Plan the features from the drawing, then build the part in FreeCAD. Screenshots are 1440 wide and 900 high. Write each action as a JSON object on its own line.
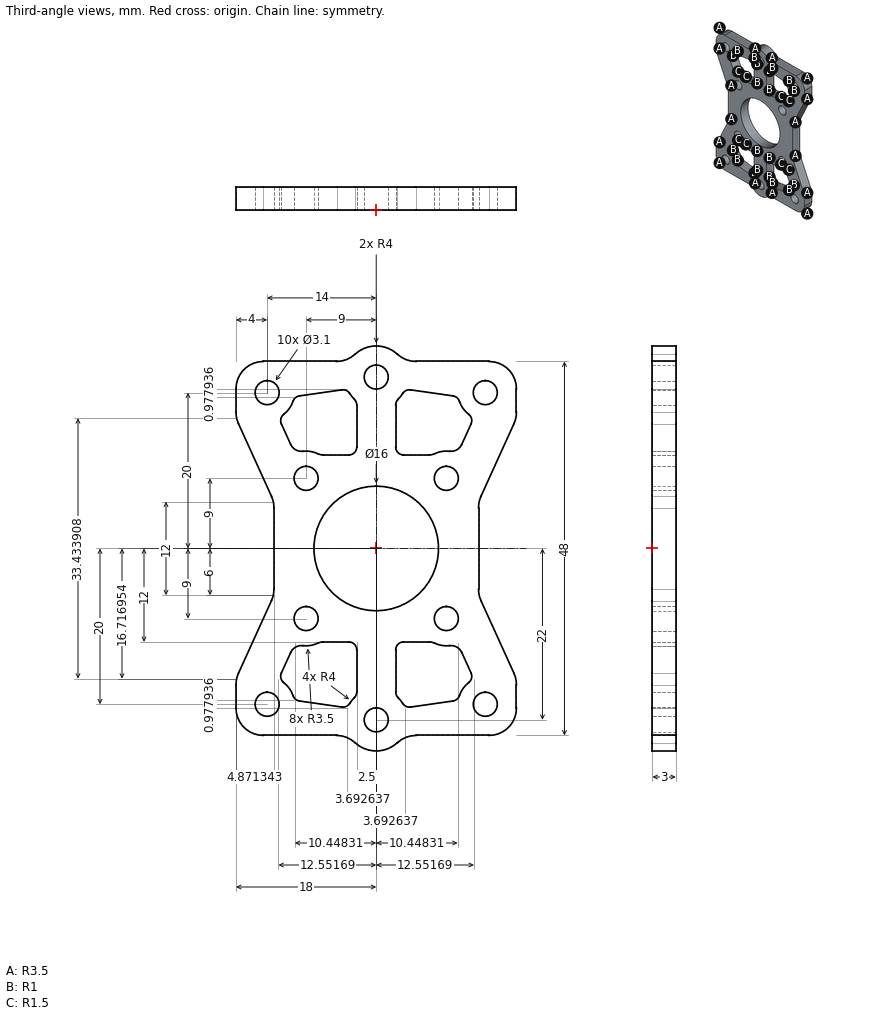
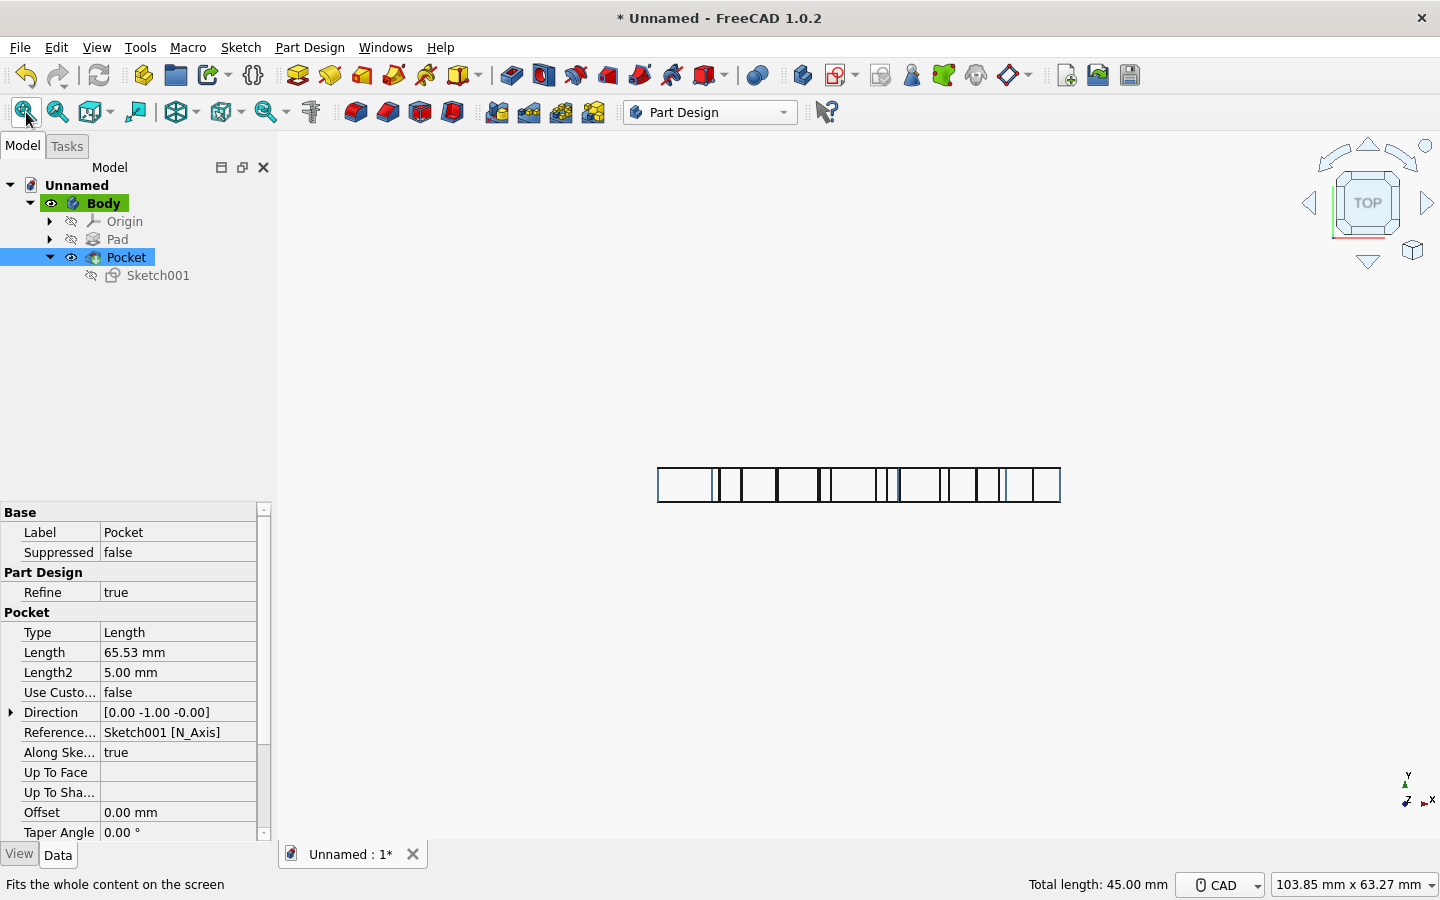
{"action": "left_click", "coordinate": [820, 484], "text": "ctrl"}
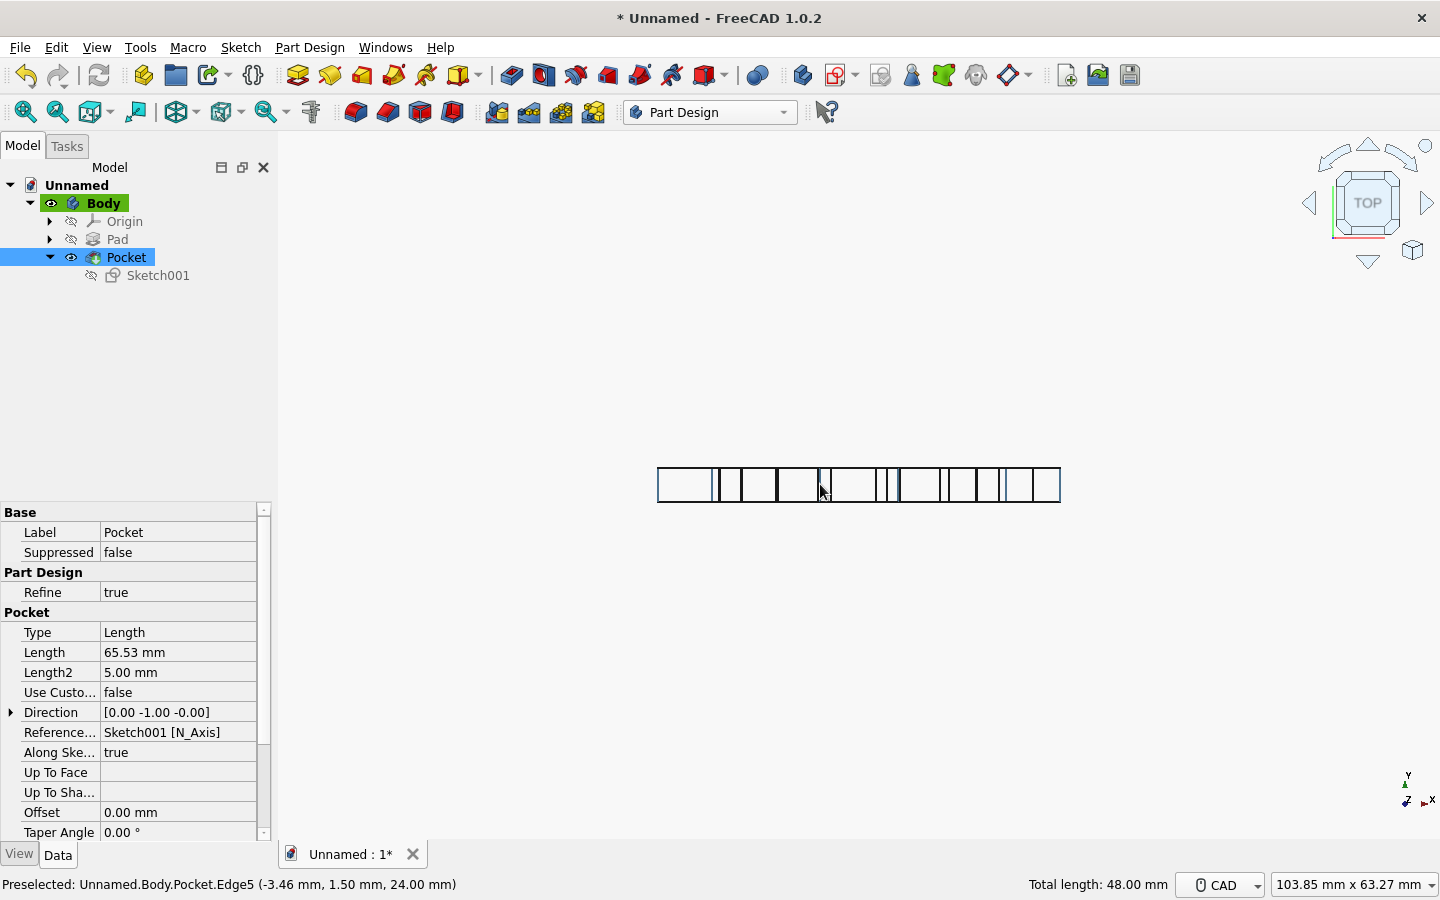
{"action": "key", "text": "v 1"}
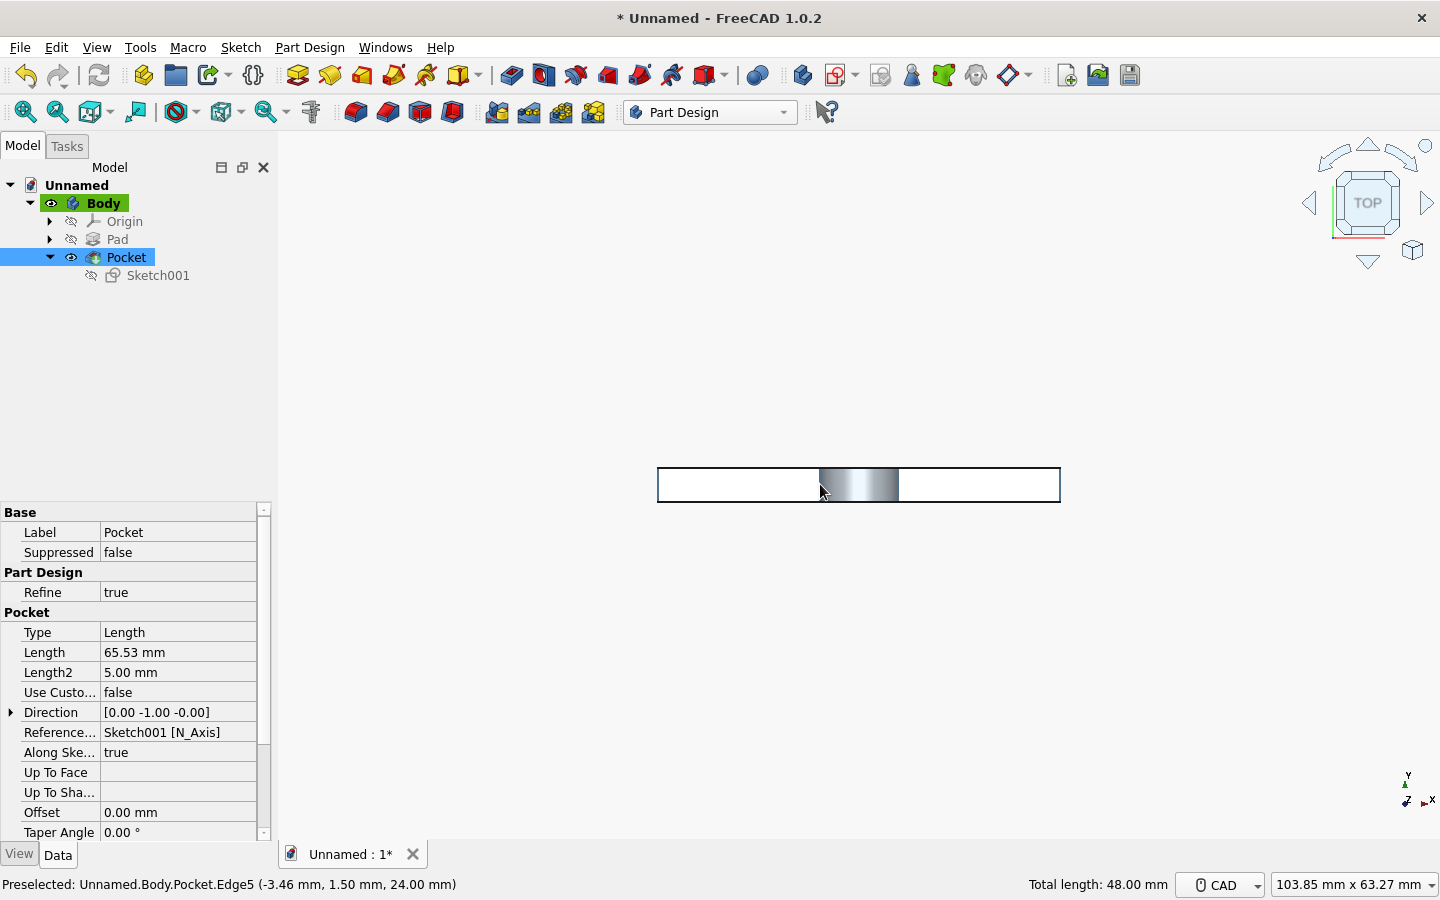
{"action": "left_click", "coordinate": [356, 112]}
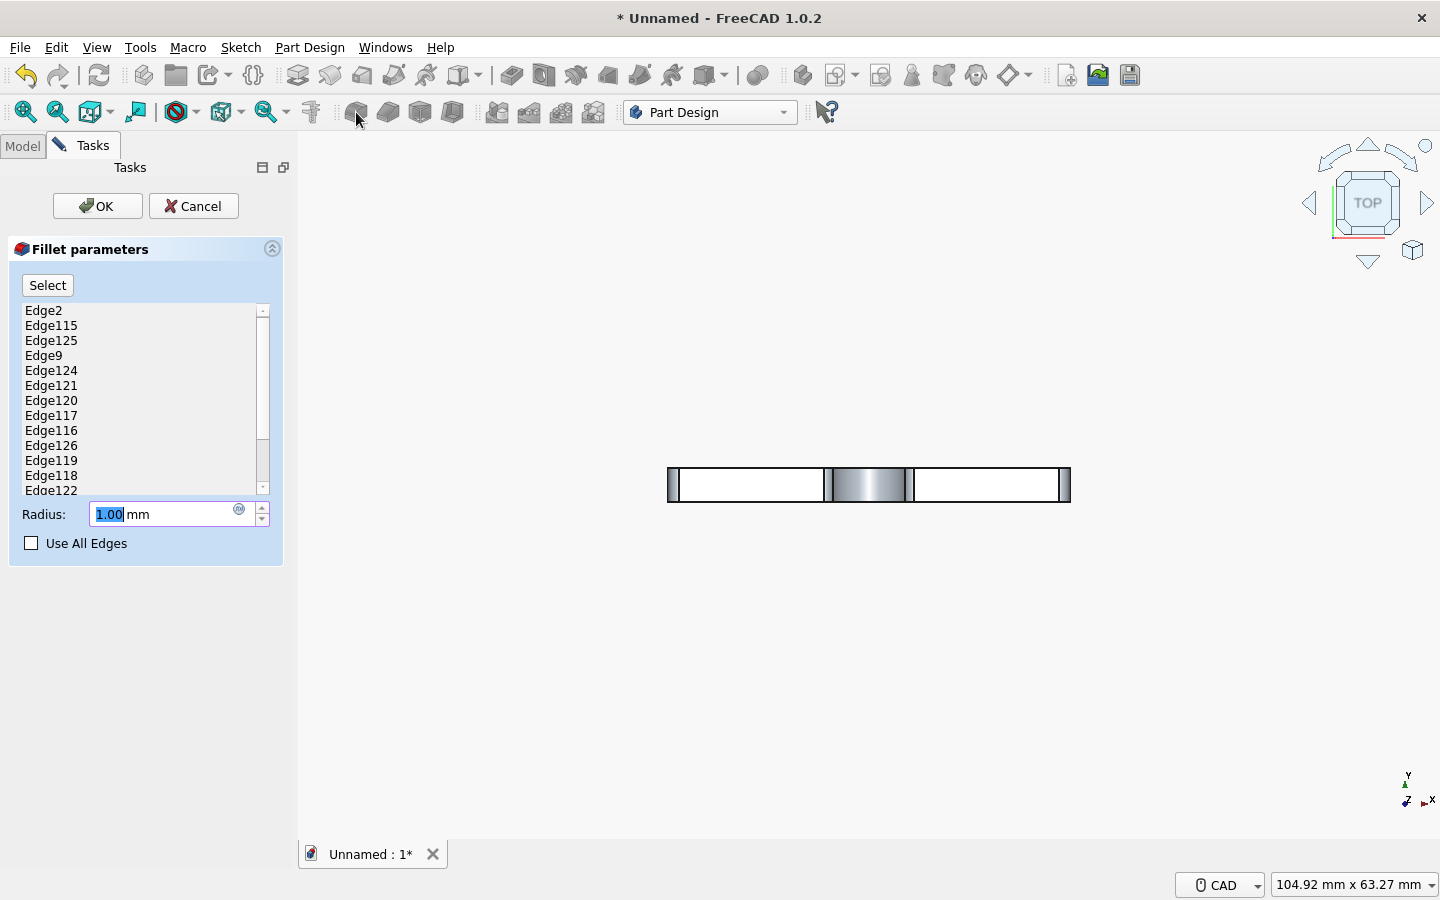
{"action": "type", "text": "3.5"}
{"action": "key", "text": "Tab"}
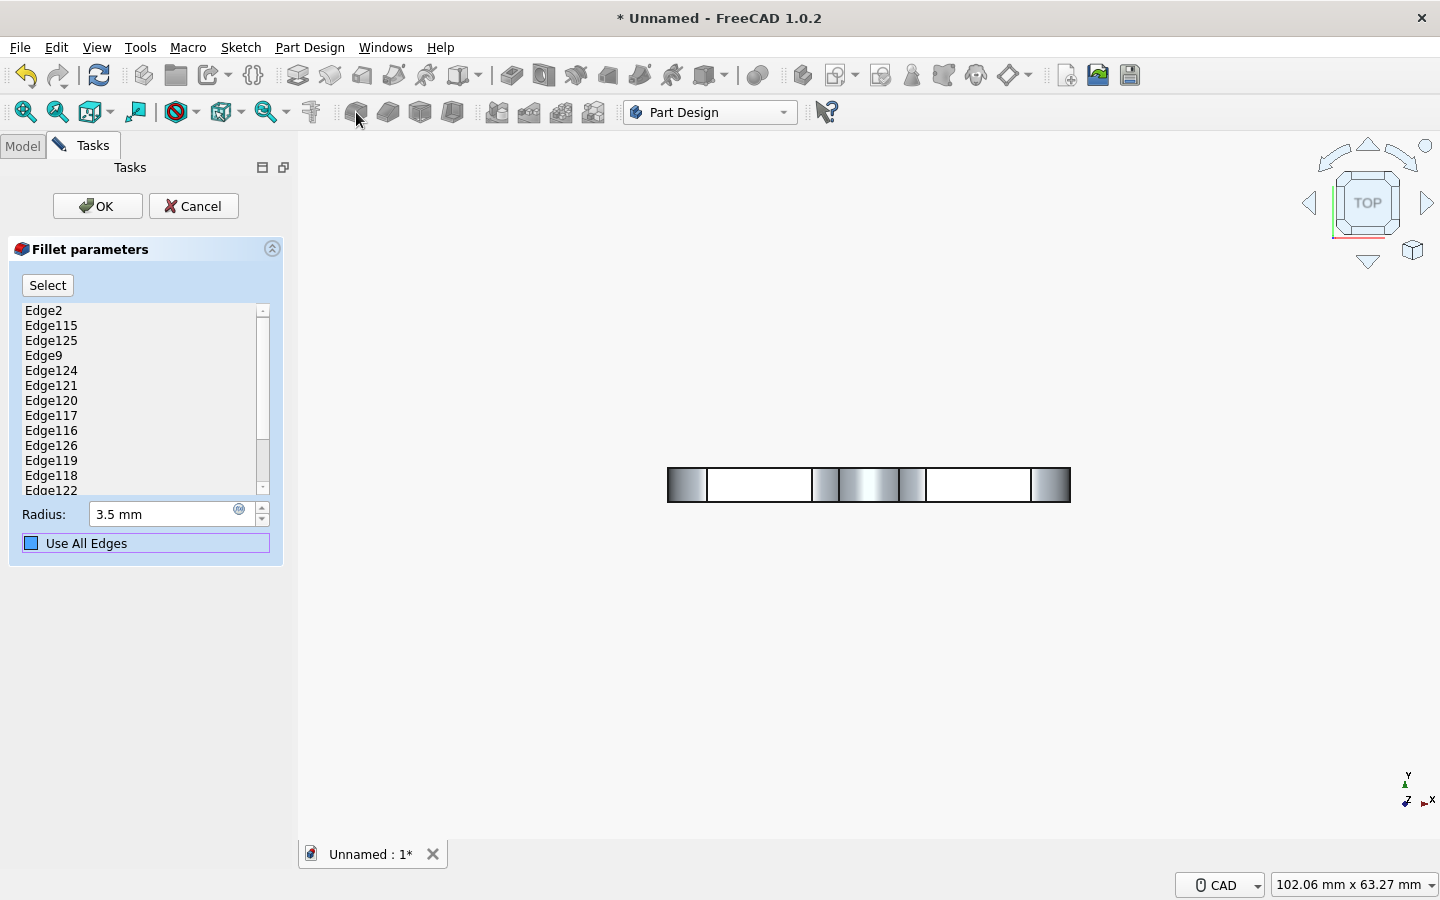
{"action": "left_click", "coordinate": [98, 206]}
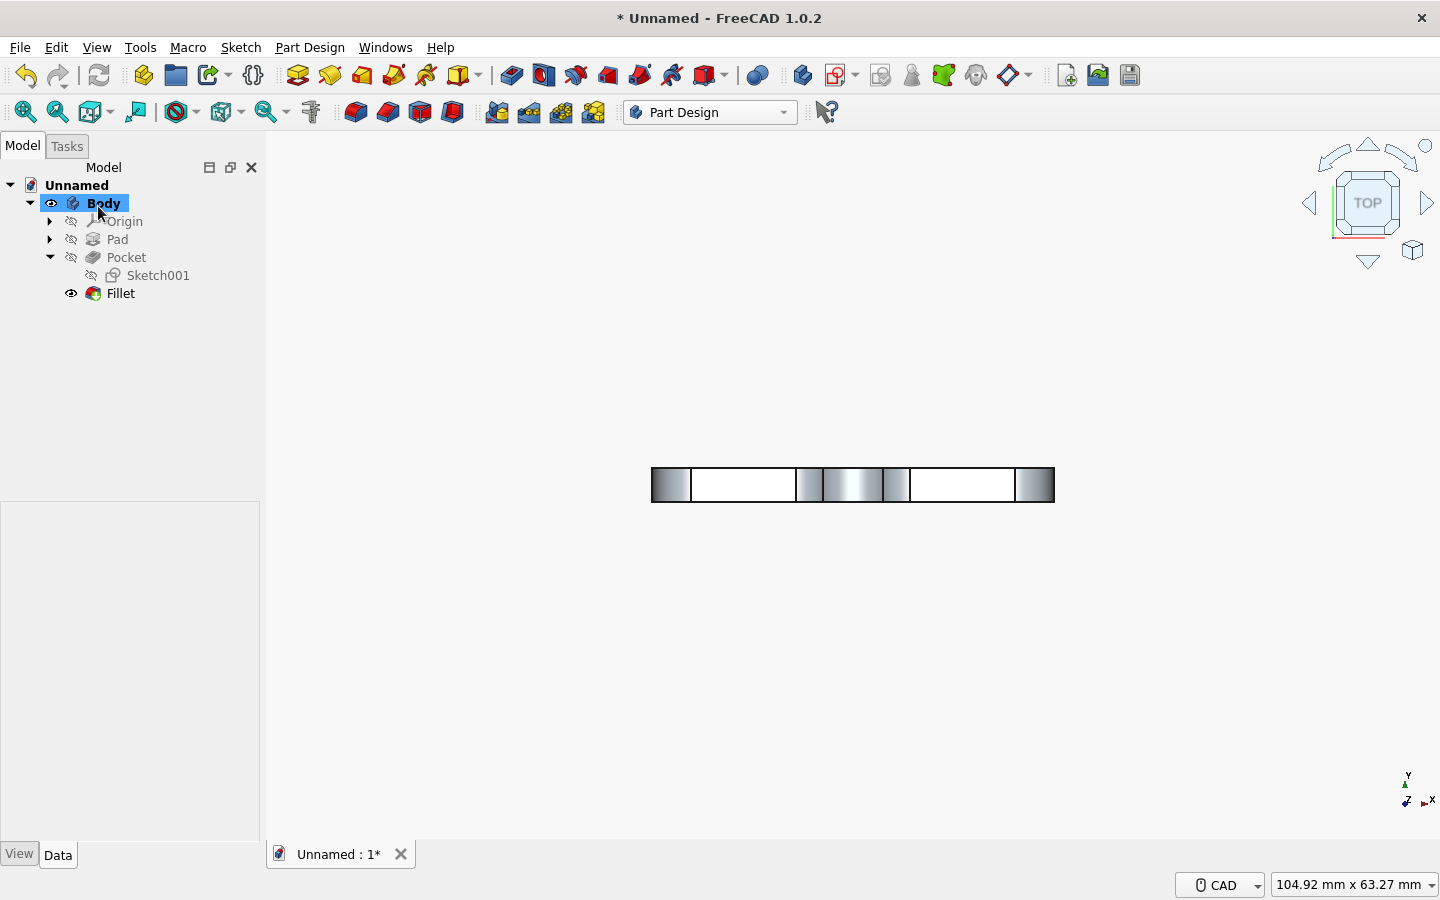
{"action": "left_click", "coordinate": [26, 112]}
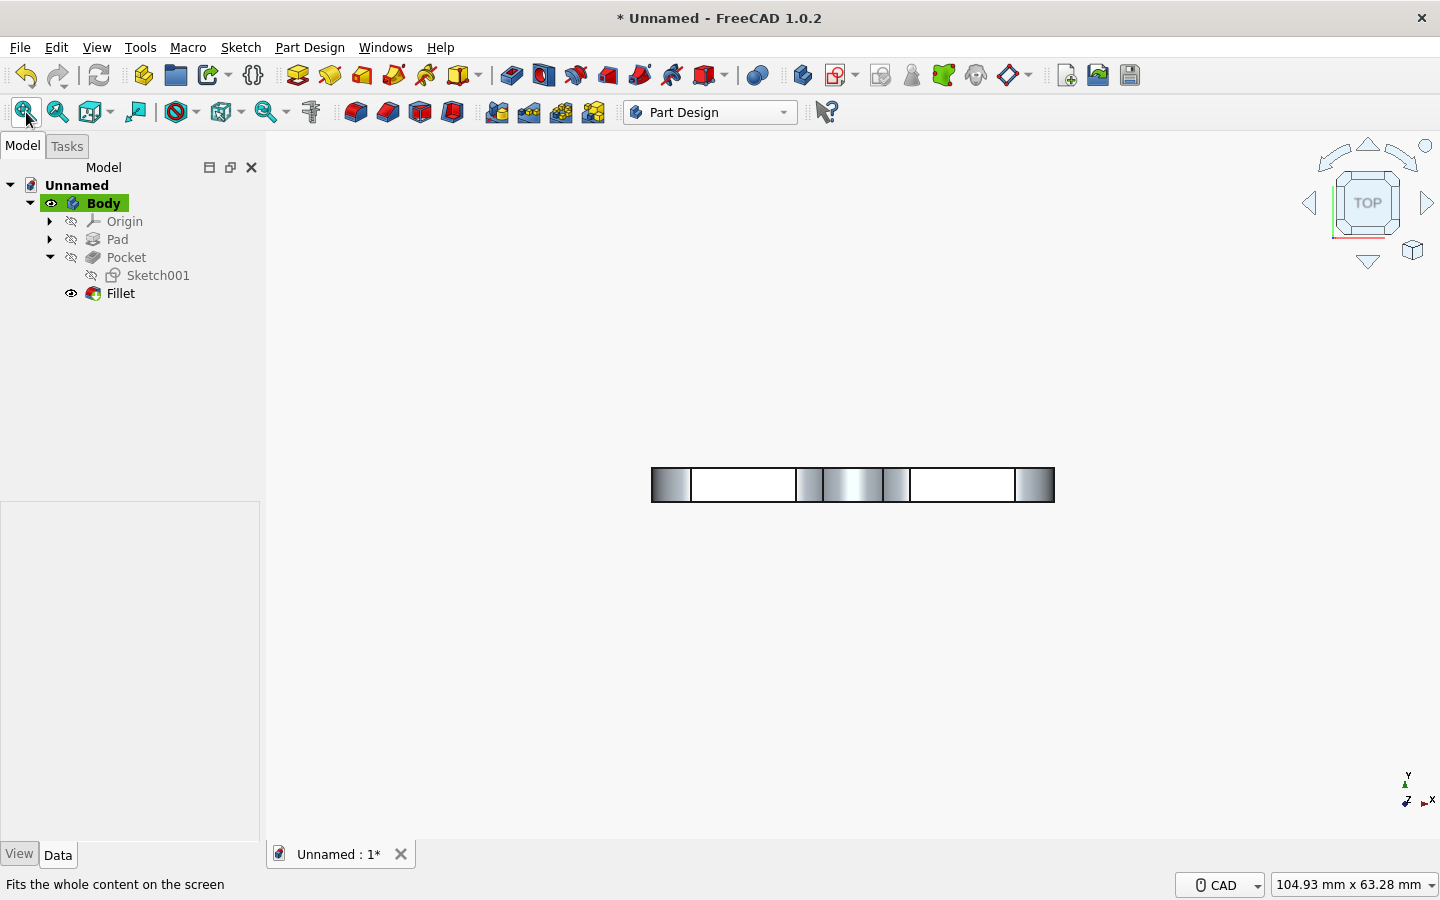
{"action": "key", "text": "0"}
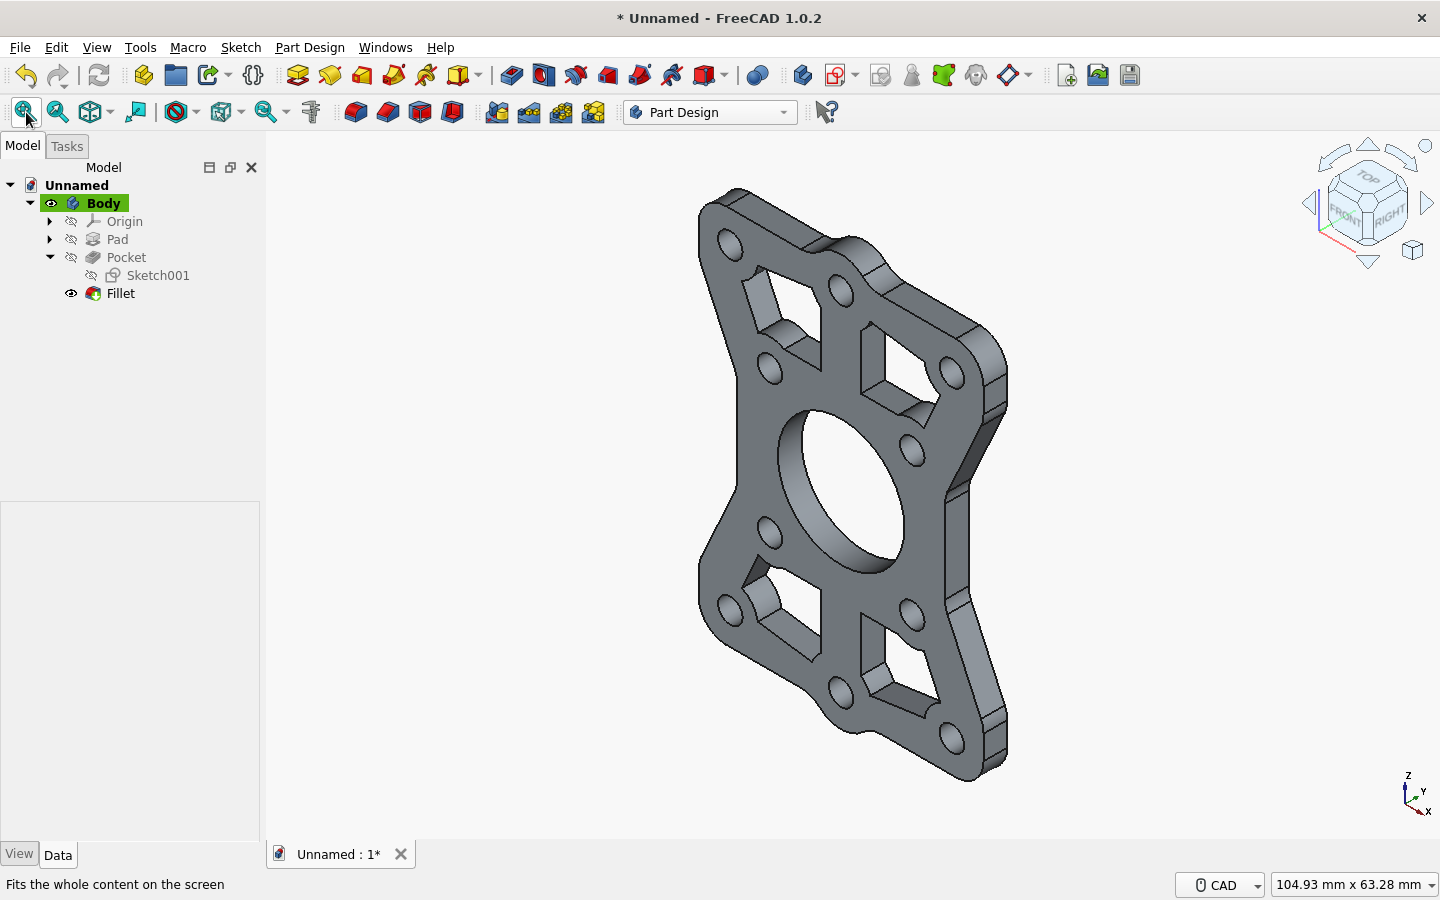
{"action": "key", "text": "2"}